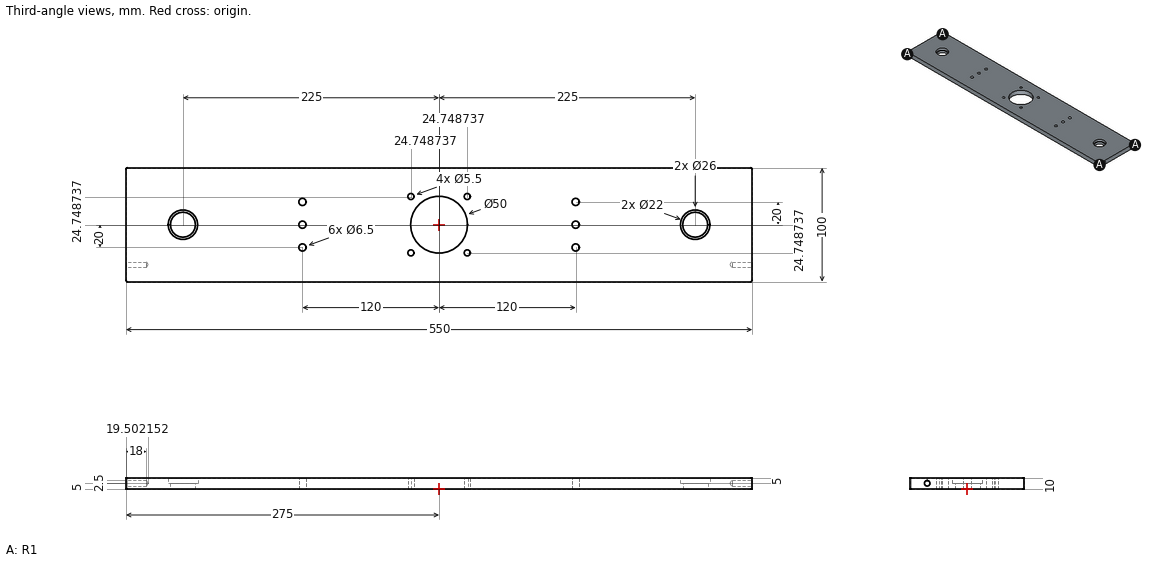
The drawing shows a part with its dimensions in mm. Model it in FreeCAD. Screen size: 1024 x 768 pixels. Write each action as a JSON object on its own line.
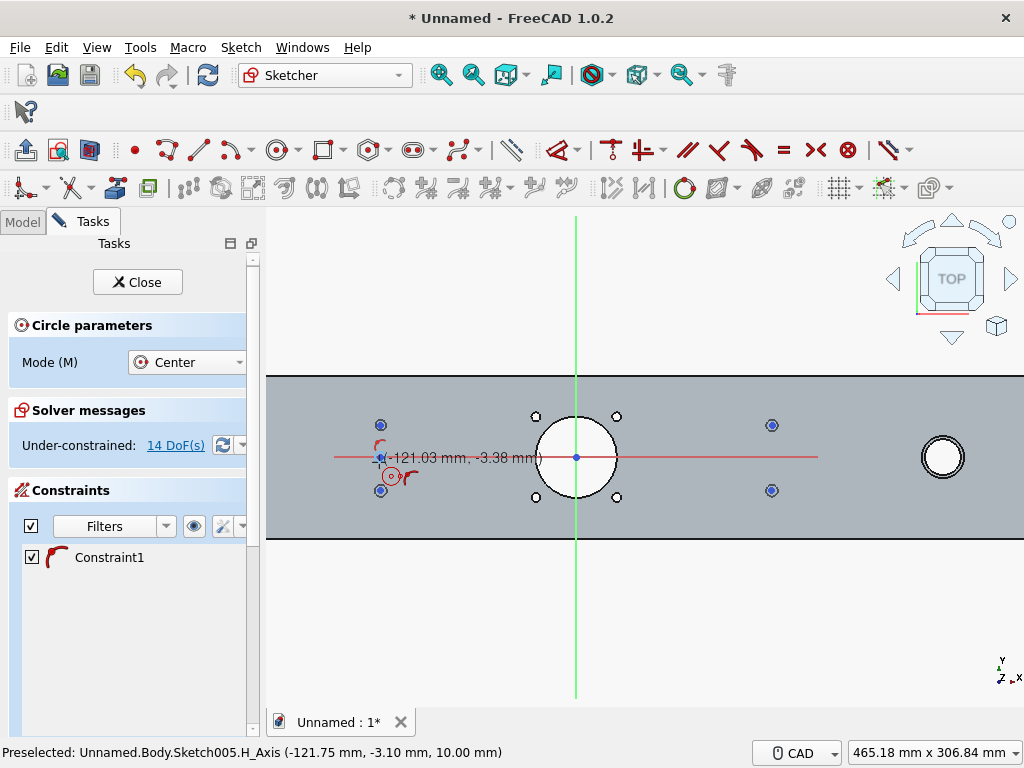
{"action": "scroll", "coordinate": [772, 457], "scroll_direction": "up", "scroll_amount": 8}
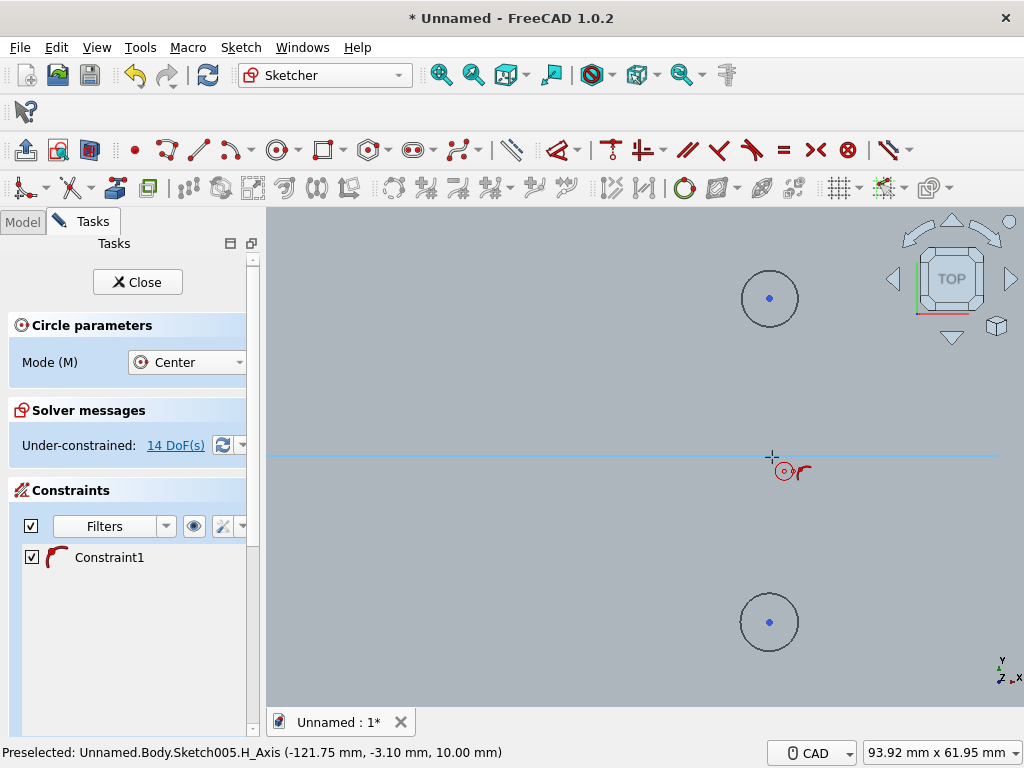
{"action": "scroll", "coordinate": [773, 457], "scroll_direction": "down", "scroll_amount": 8}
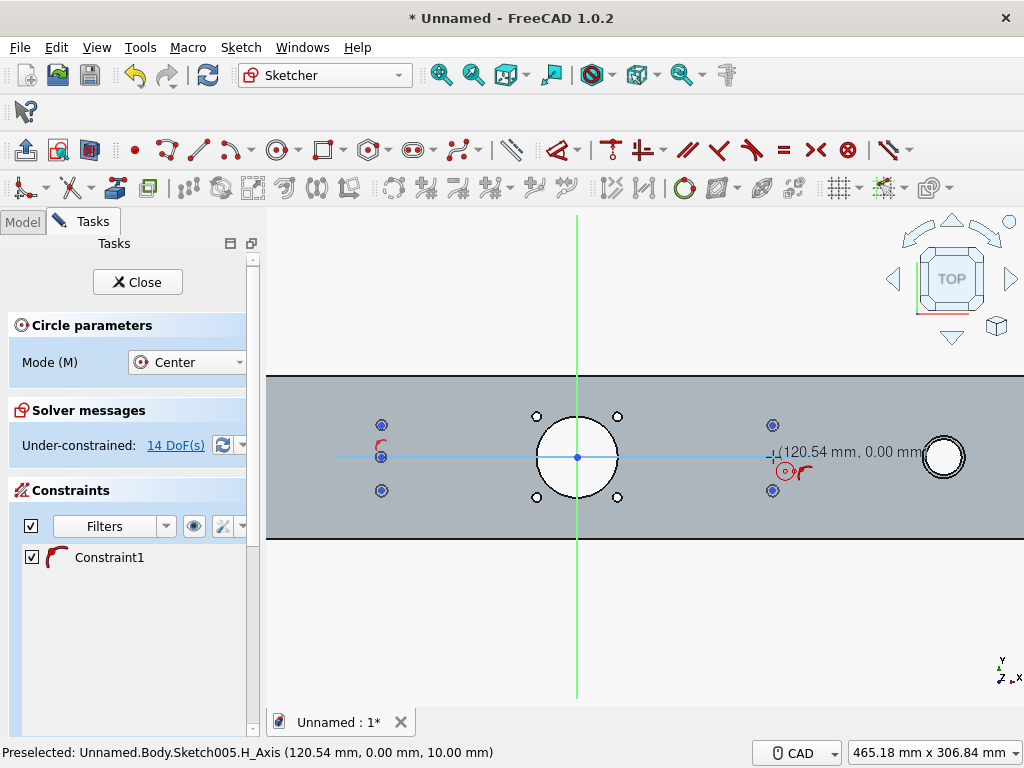
{"action": "left_click", "coordinate": [773, 457]}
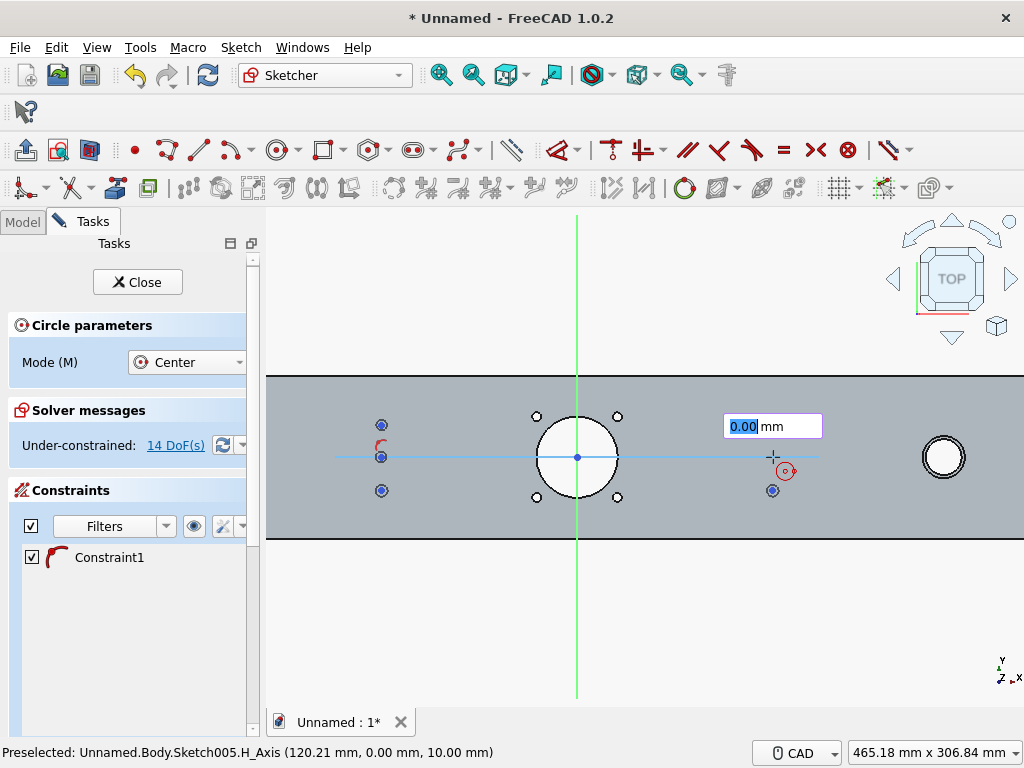
{"action": "scroll", "coordinate": [771, 462], "scroll_direction": "up", "scroll_amount": 6}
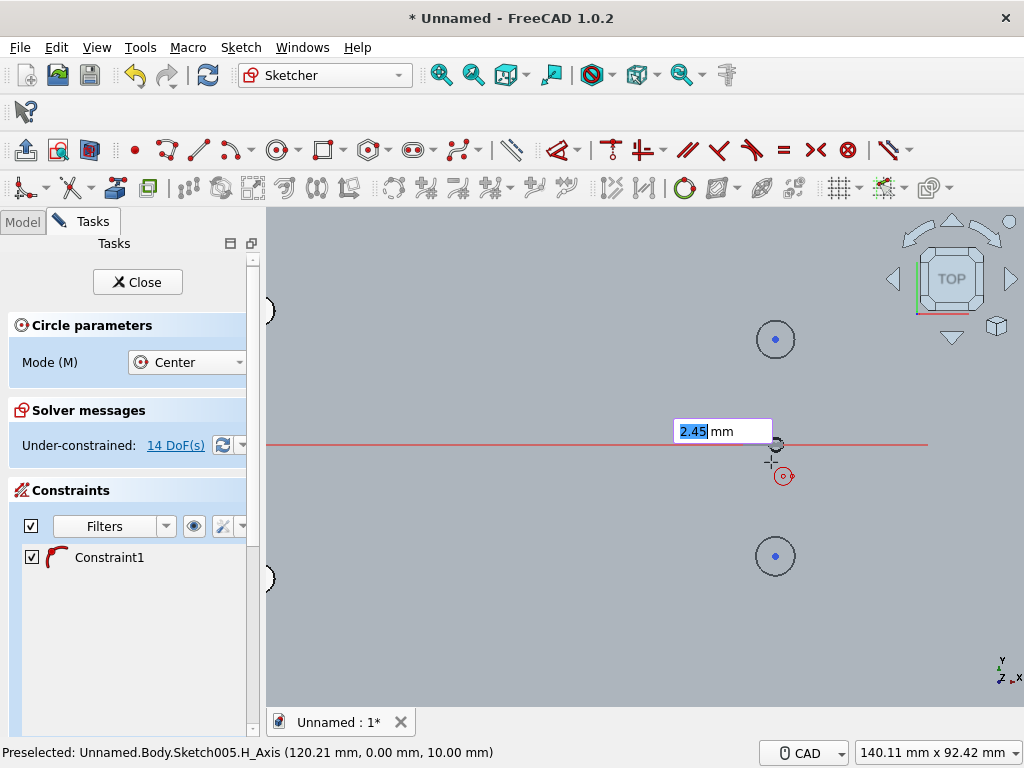
{"action": "left_click", "coordinate": [769, 461]}
{"action": "key", "text": "Escape"}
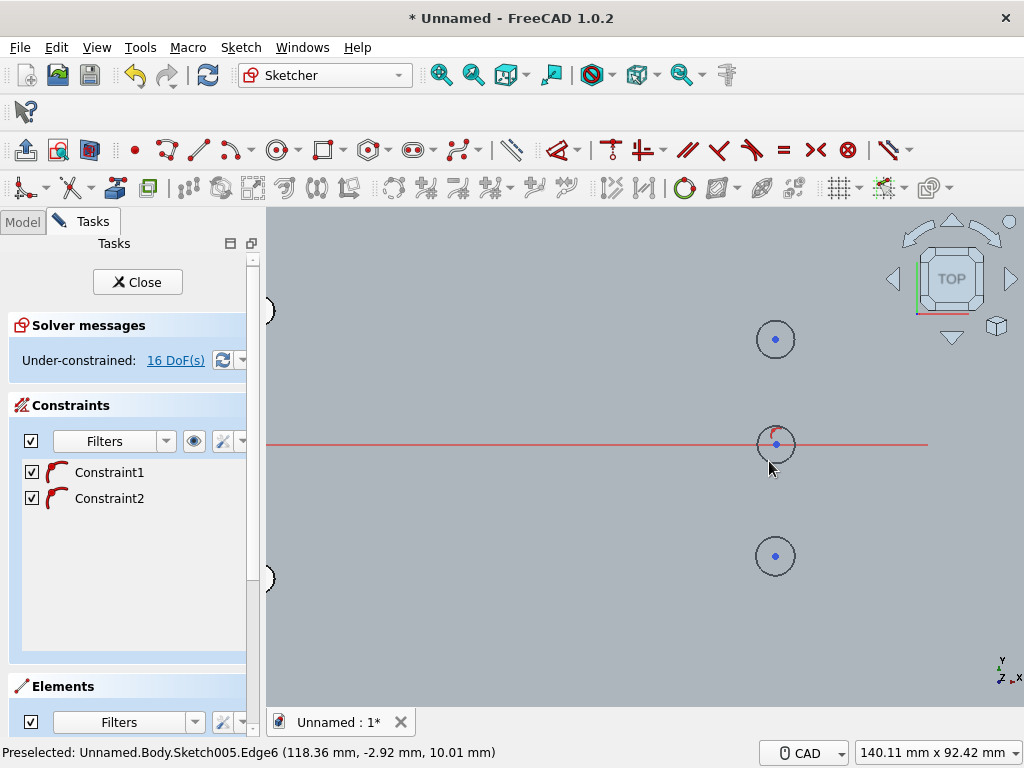
{"action": "scroll", "coordinate": [771, 462], "scroll_direction": "down", "scroll_amount": 6}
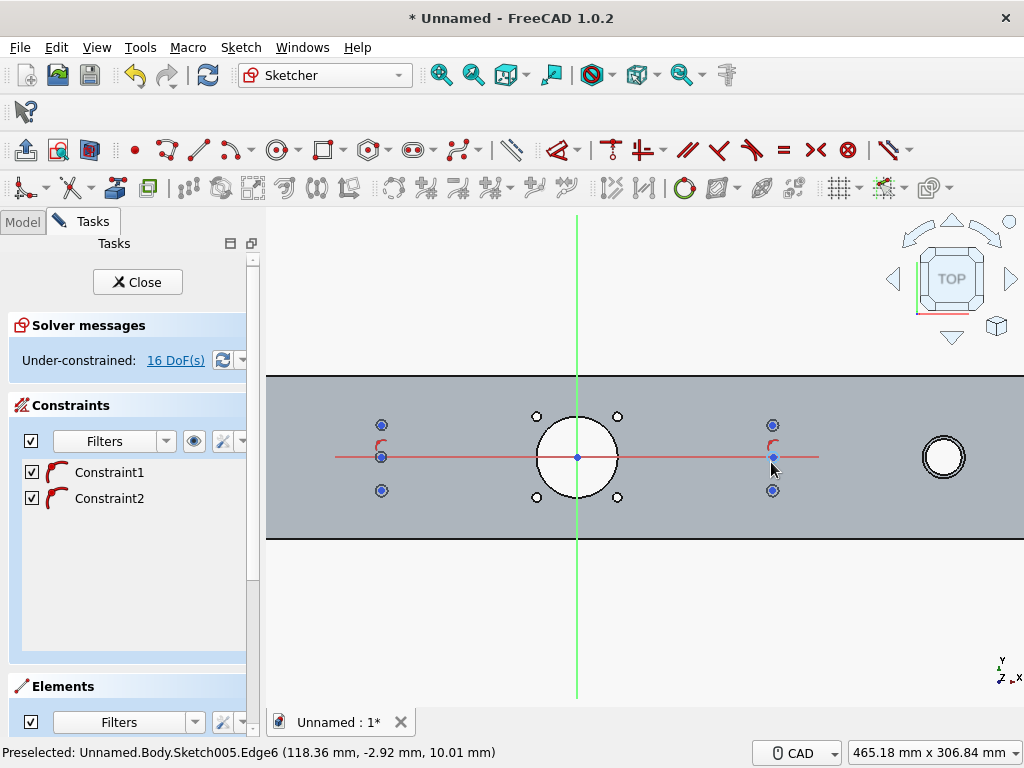
{"action": "scroll", "coordinate": [386, 487], "scroll_direction": "up", "scroll_amount": 5}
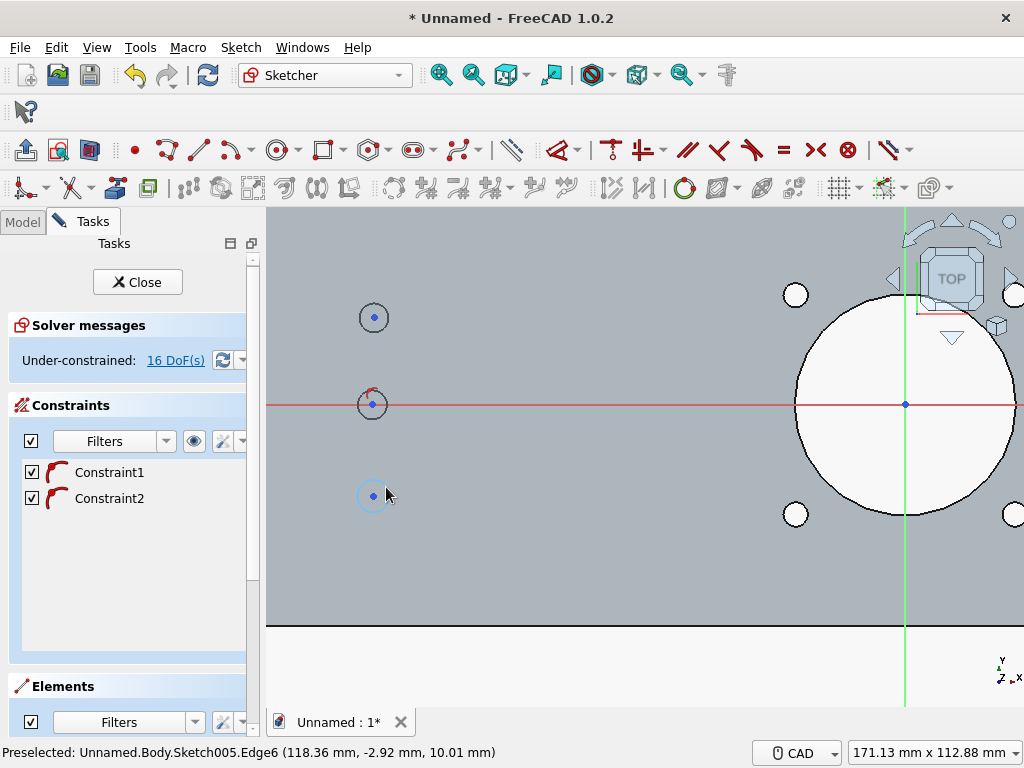
{"action": "left_click", "coordinate": [385, 485]}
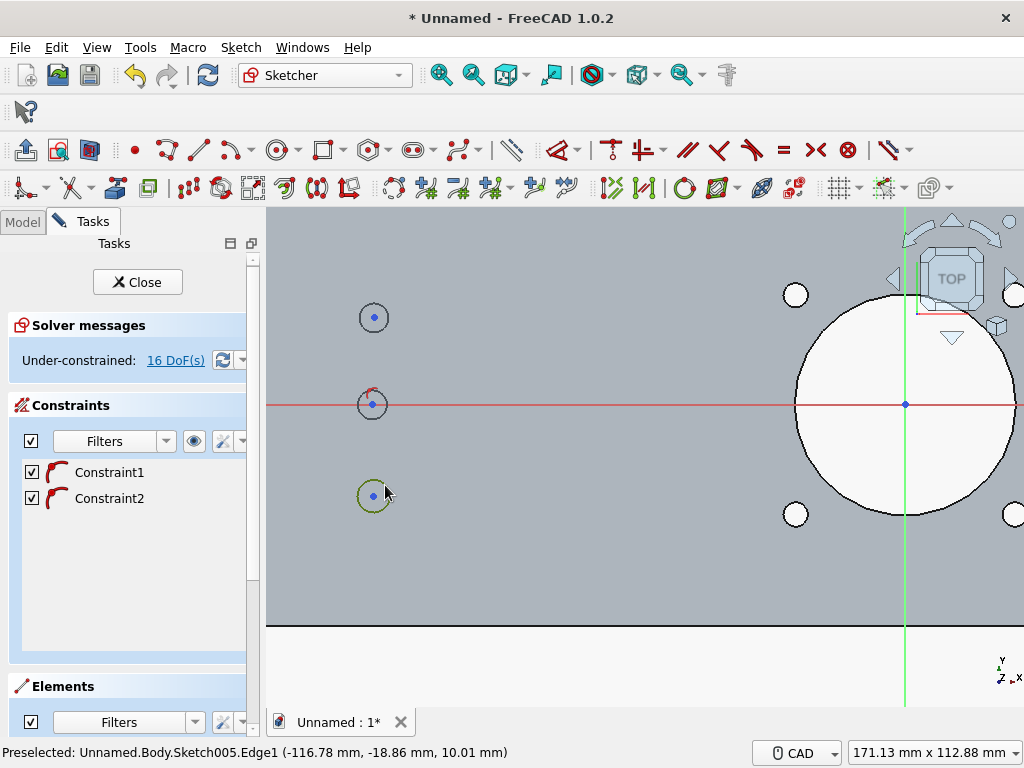
{"action": "scroll", "coordinate": [385, 487], "scroll_direction": "down", "scroll_amount": 5}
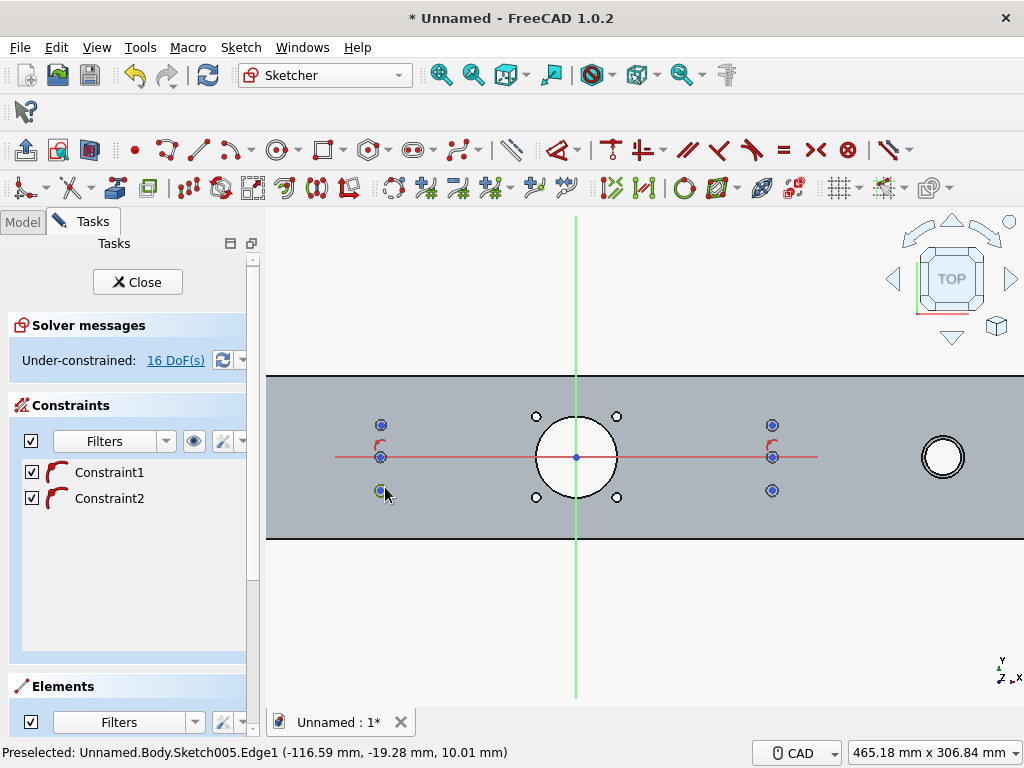
{"action": "scroll", "coordinate": [776, 487], "scroll_direction": "up", "scroll_amount": 5}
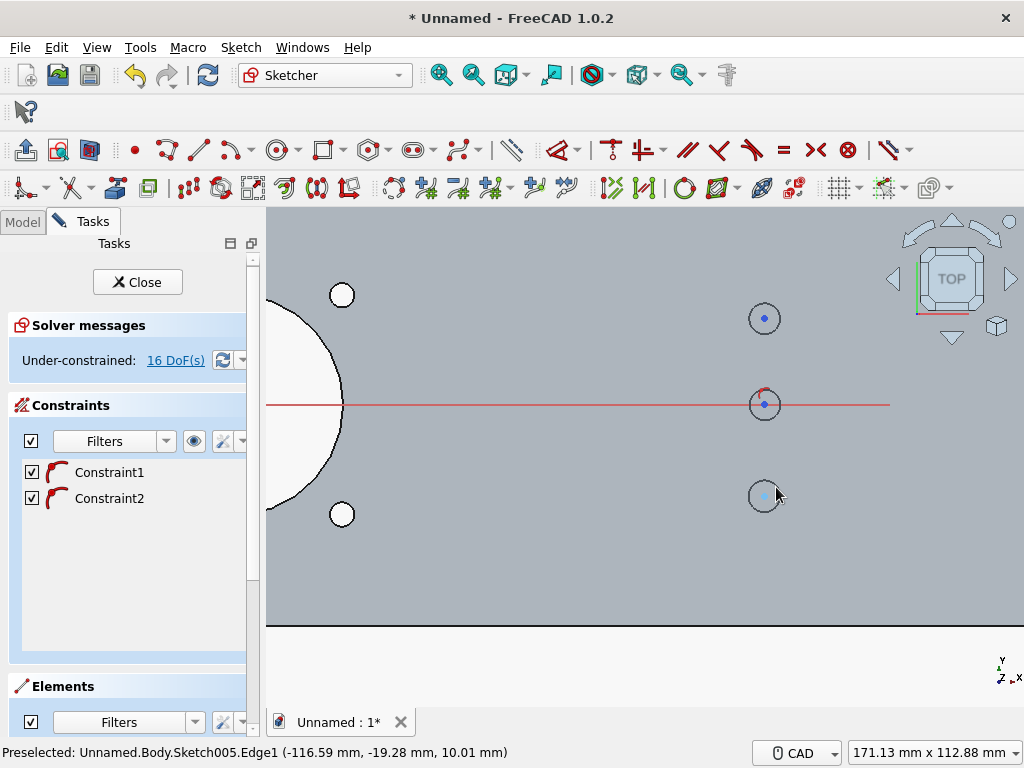
{"action": "left_click", "coordinate": [776, 485]}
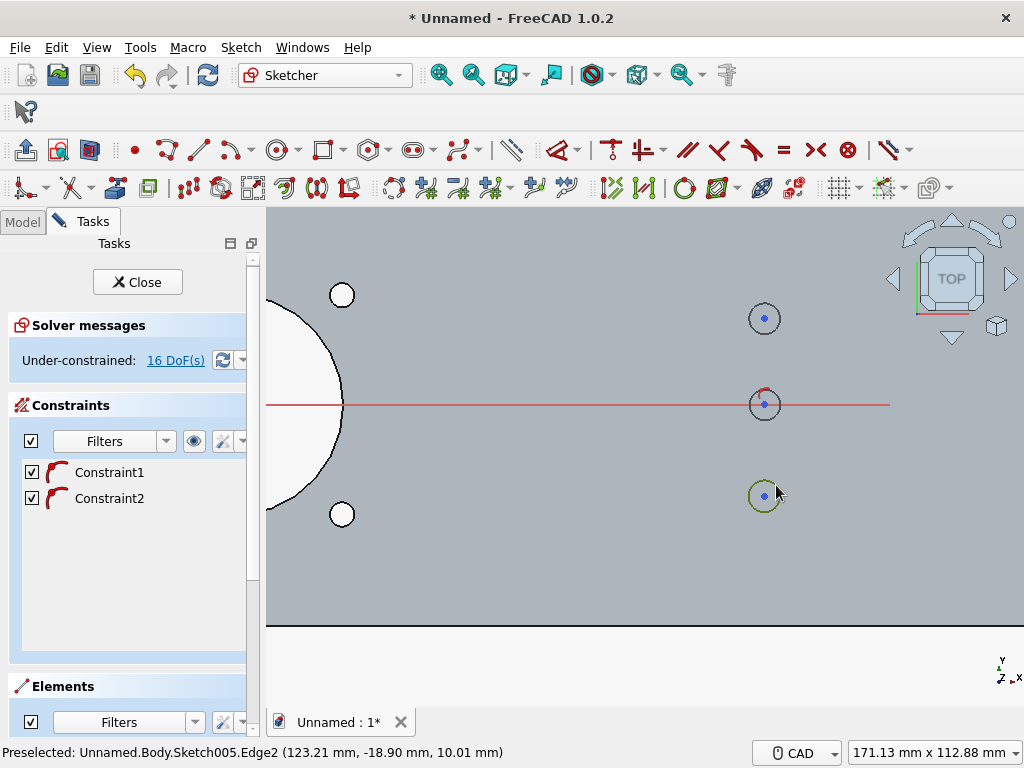
{"action": "left_click", "coordinate": [776, 308]}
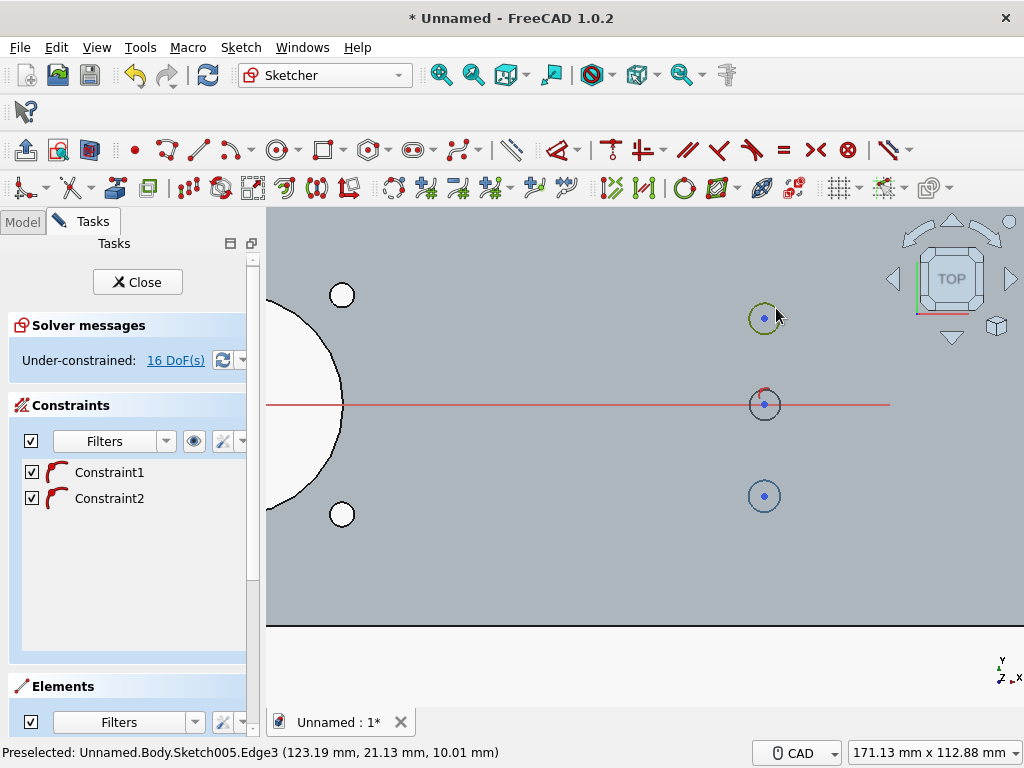
{"action": "scroll", "coordinate": [777, 487], "scroll_direction": "down", "scroll_amount": 5}